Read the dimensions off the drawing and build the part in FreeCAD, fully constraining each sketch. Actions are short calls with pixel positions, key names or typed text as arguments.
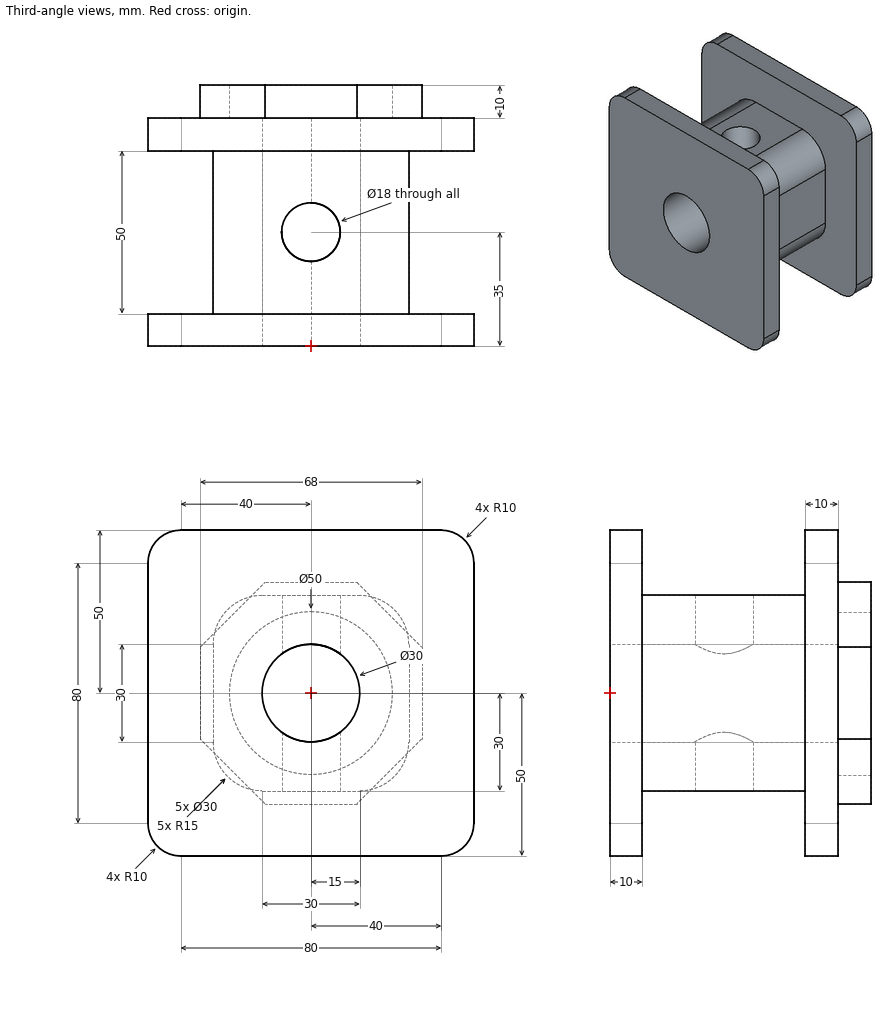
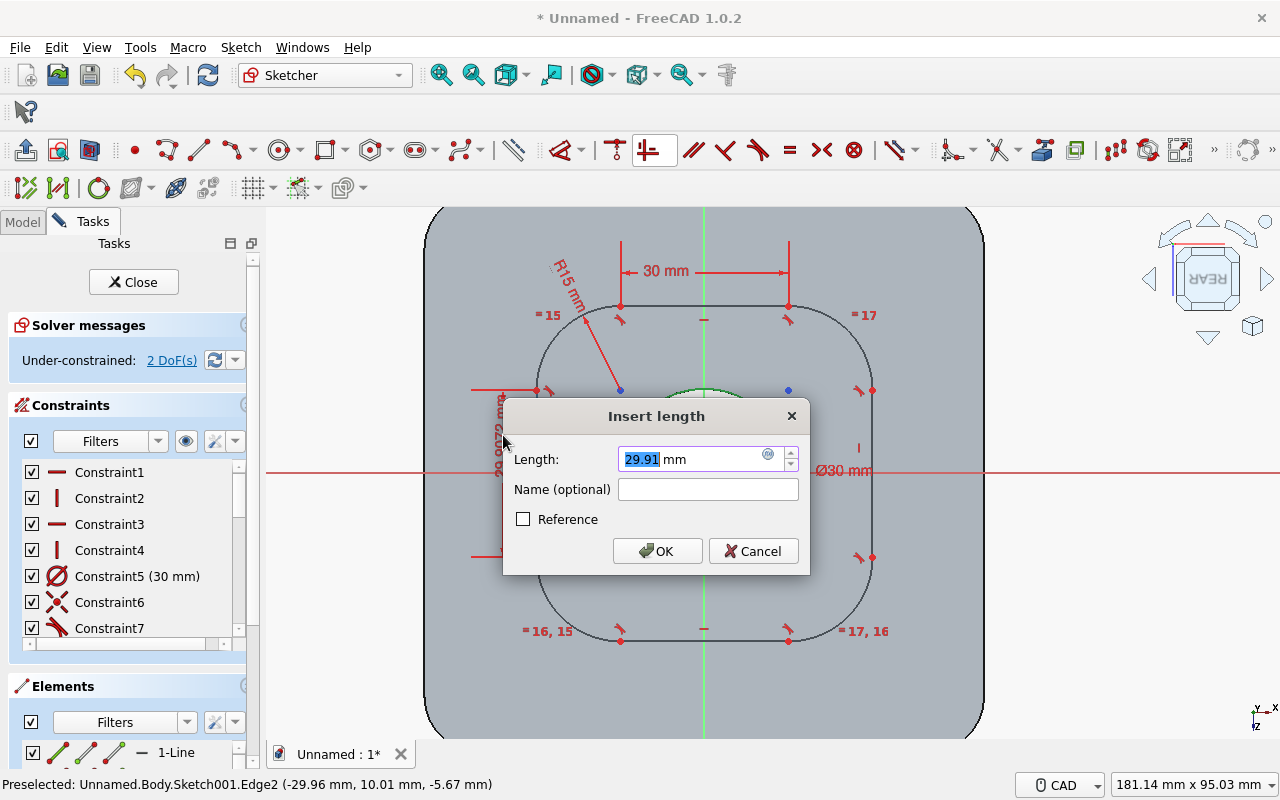
text(30)
key(Return)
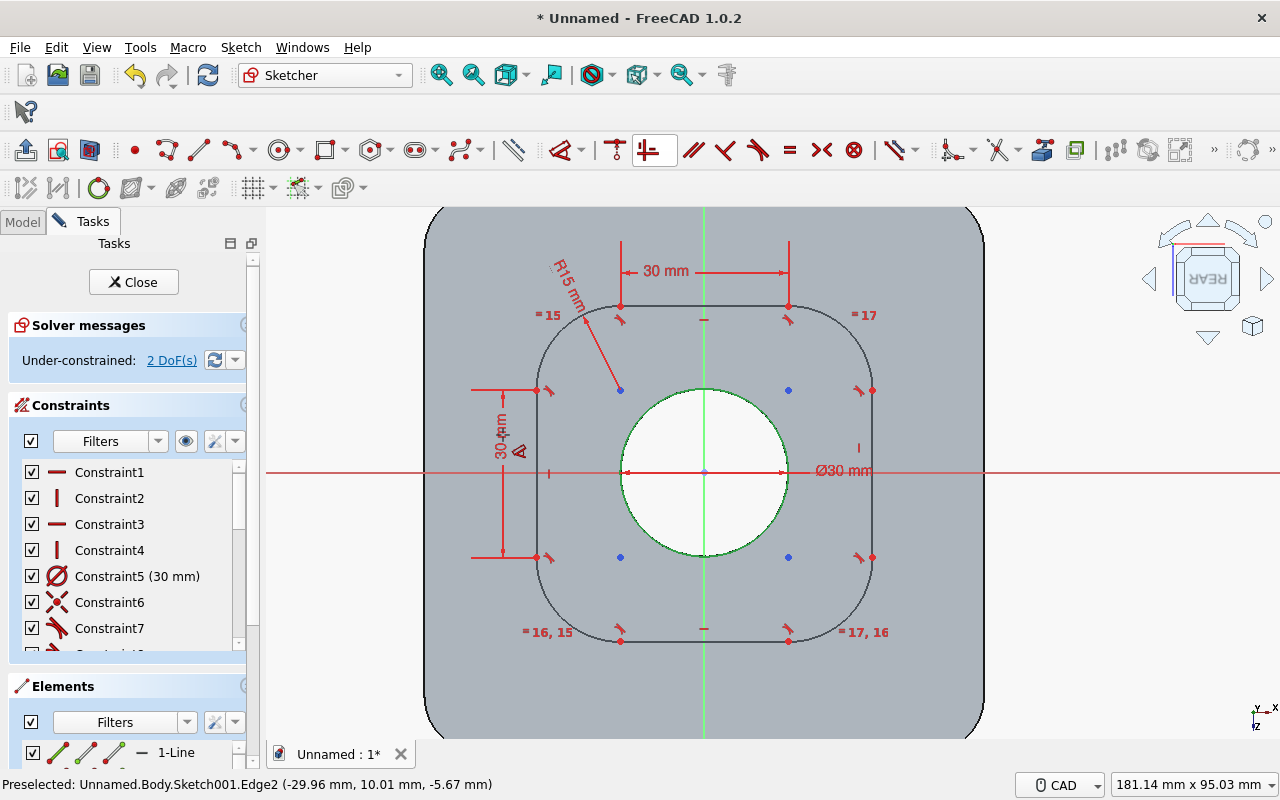
click(789, 306)
click(746, 272)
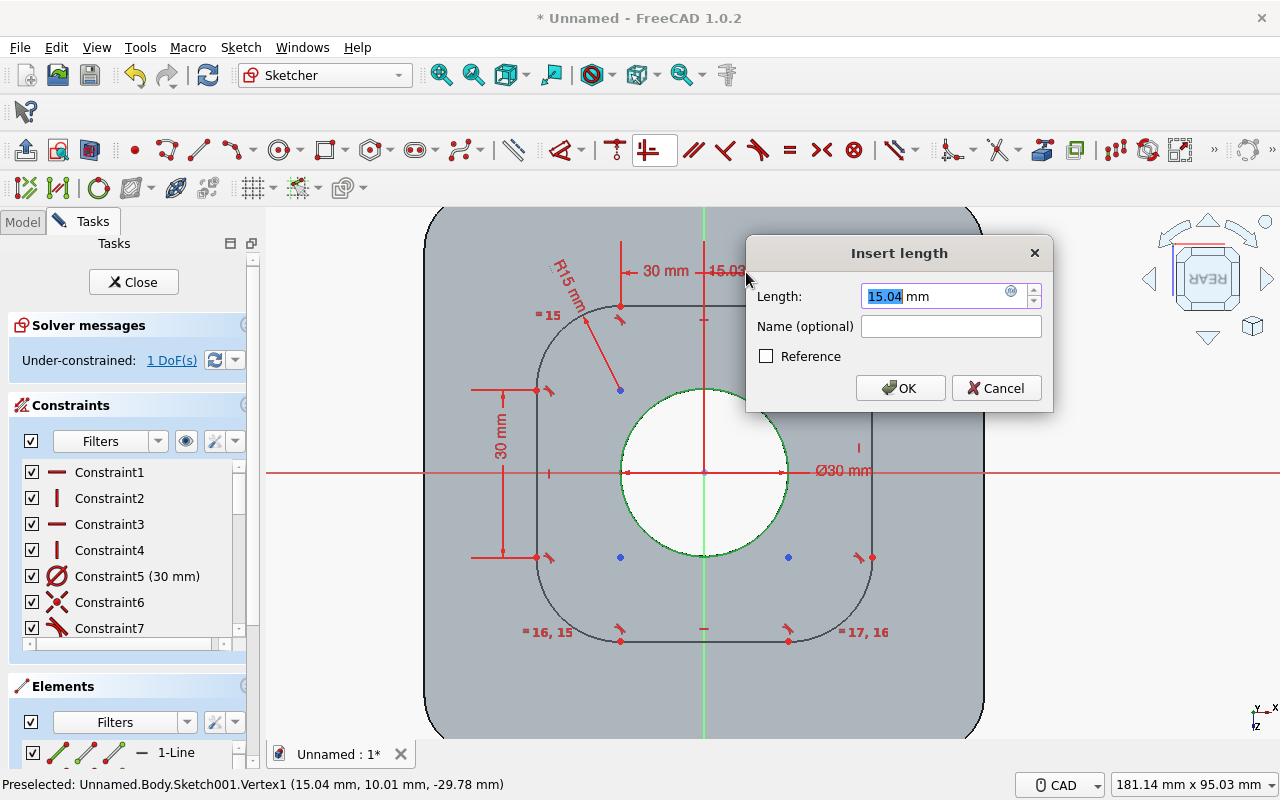
text(15)
key(Return)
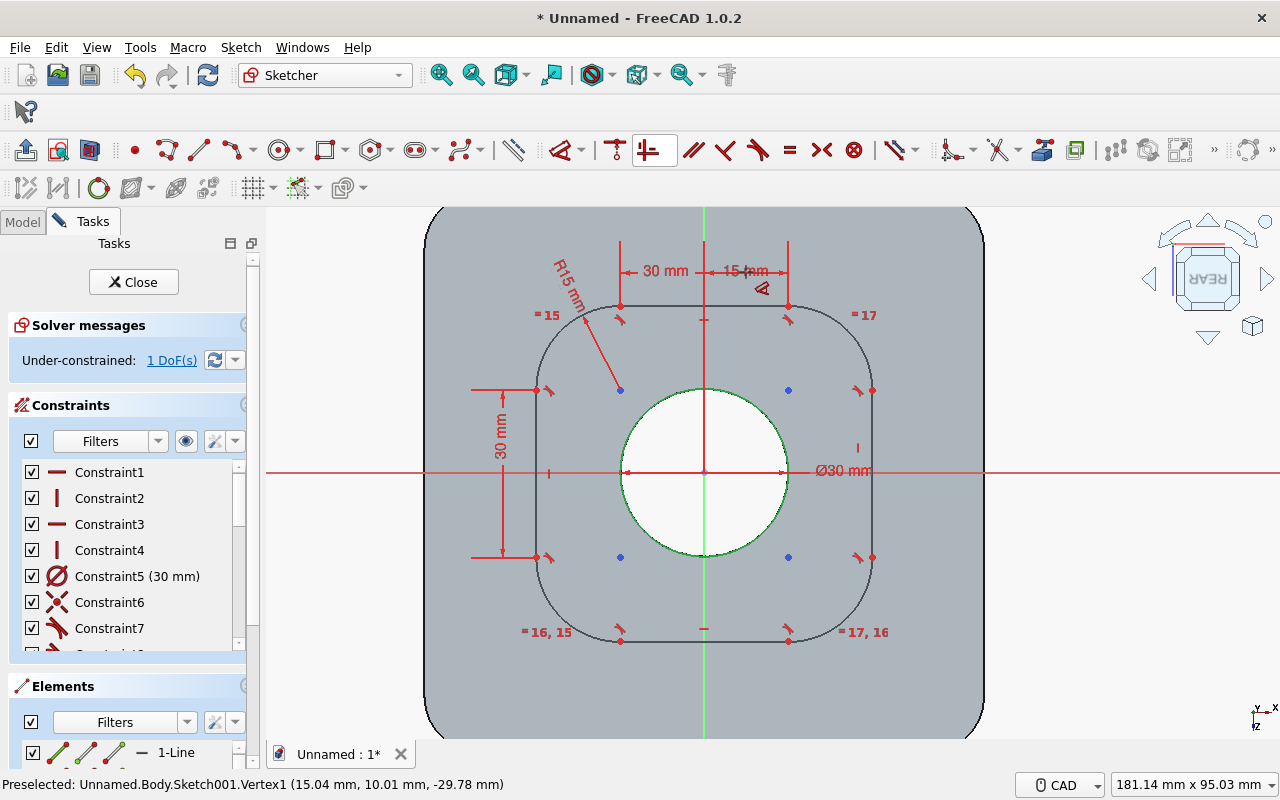
click(788, 306)
click(822, 389)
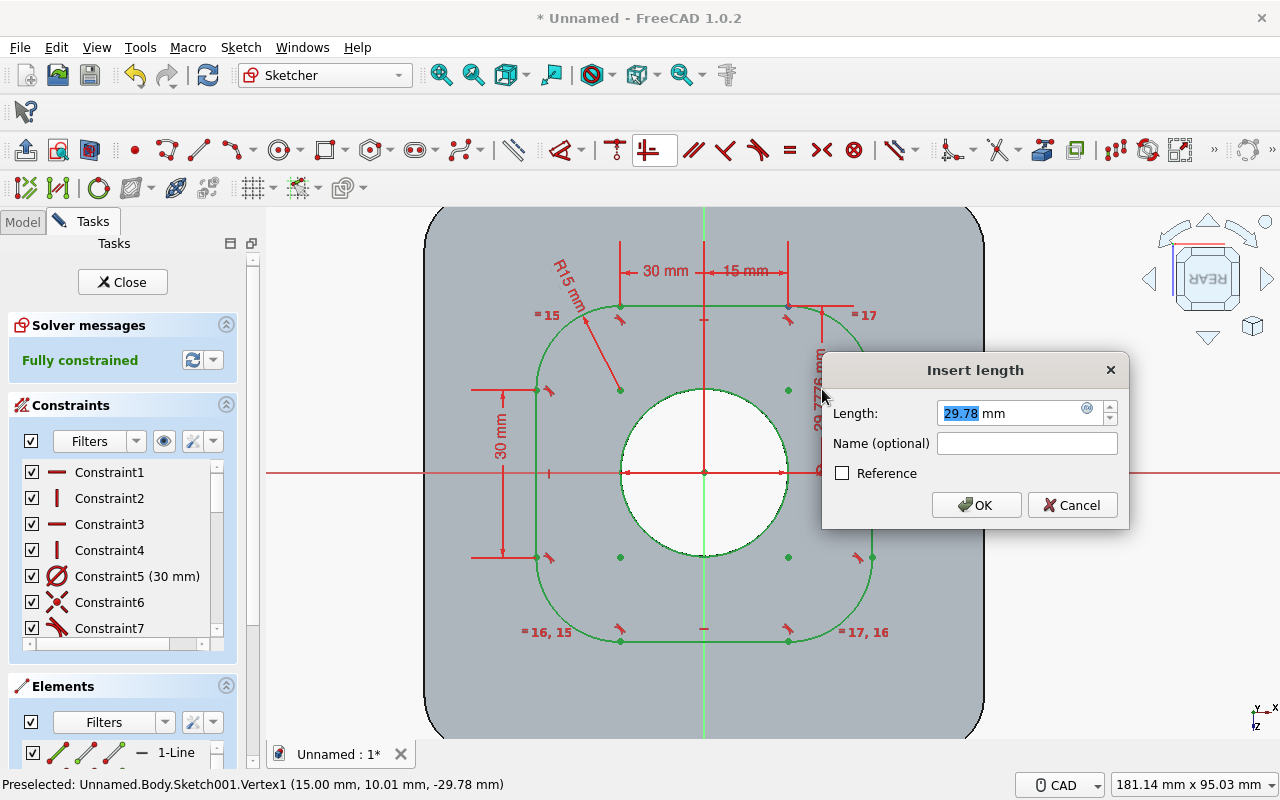
text(30)
key(Return)
key(Escape)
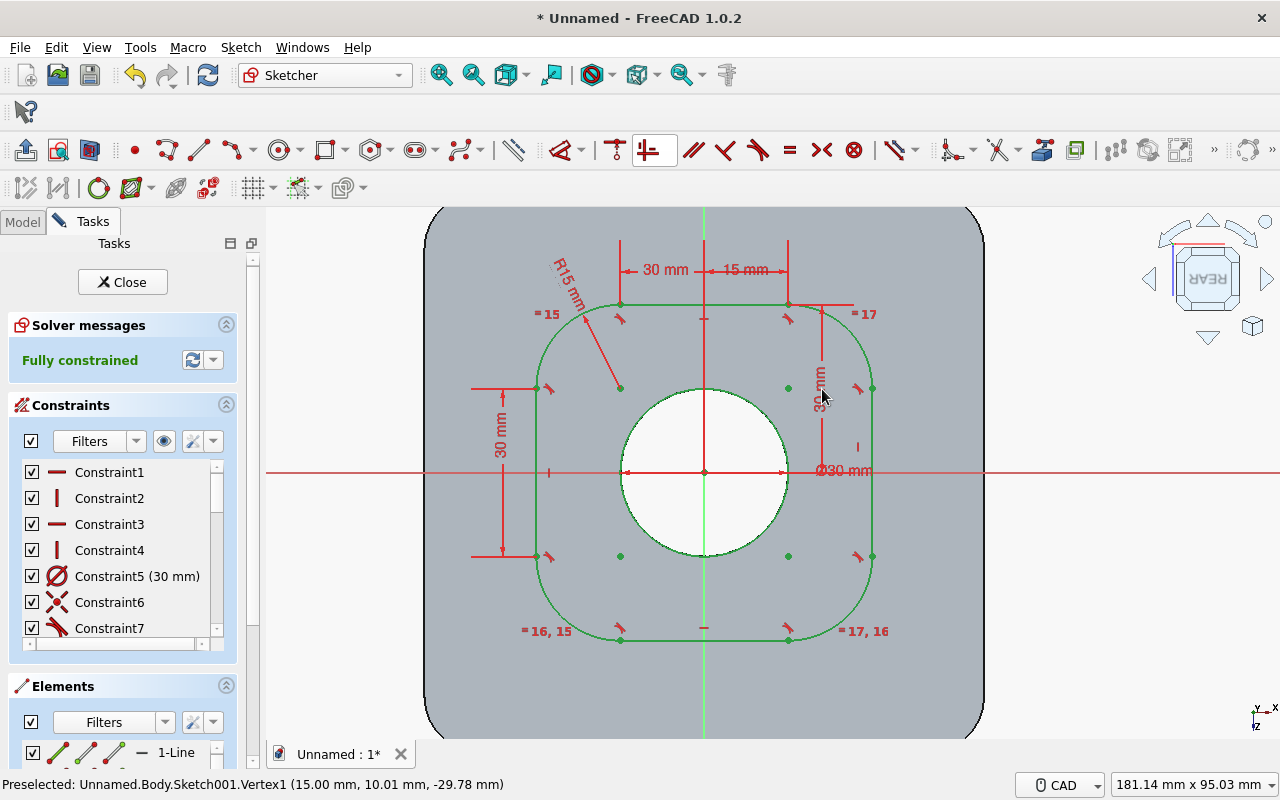
click(123, 282)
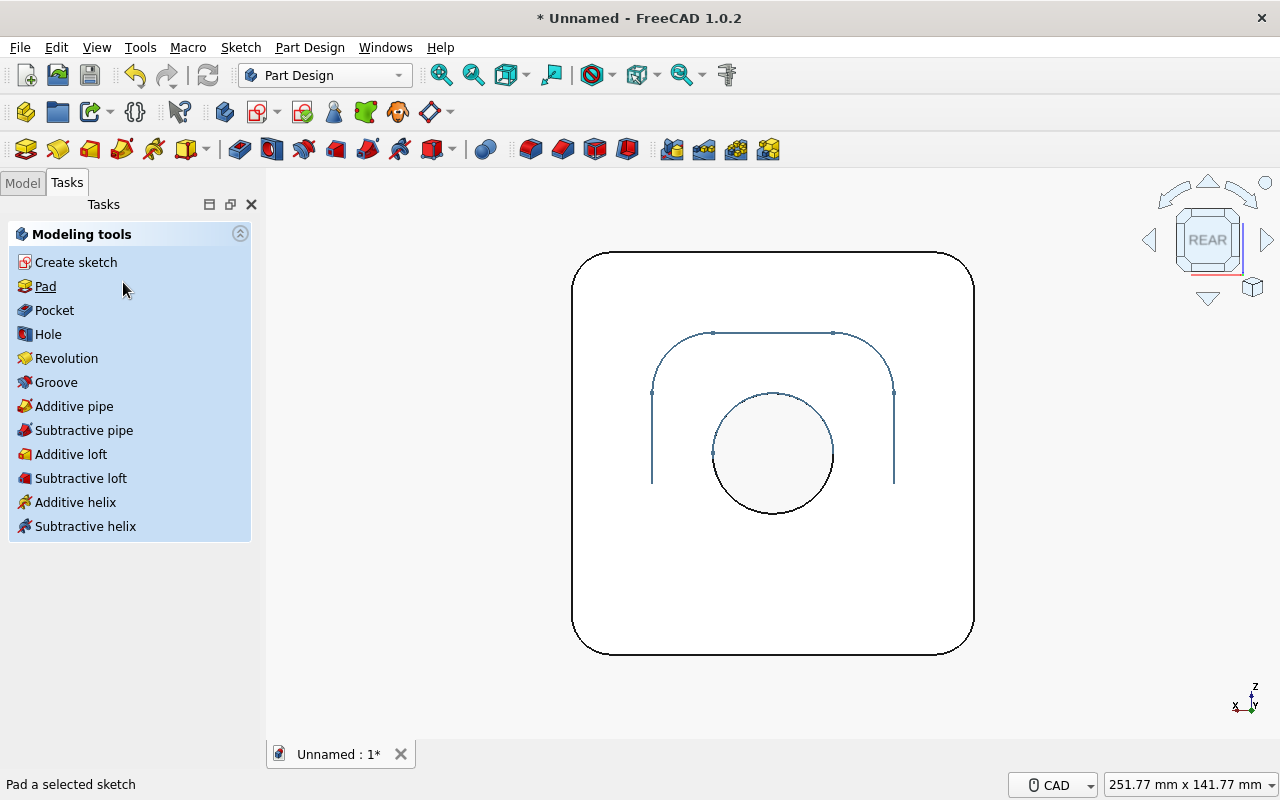
click(26, 150)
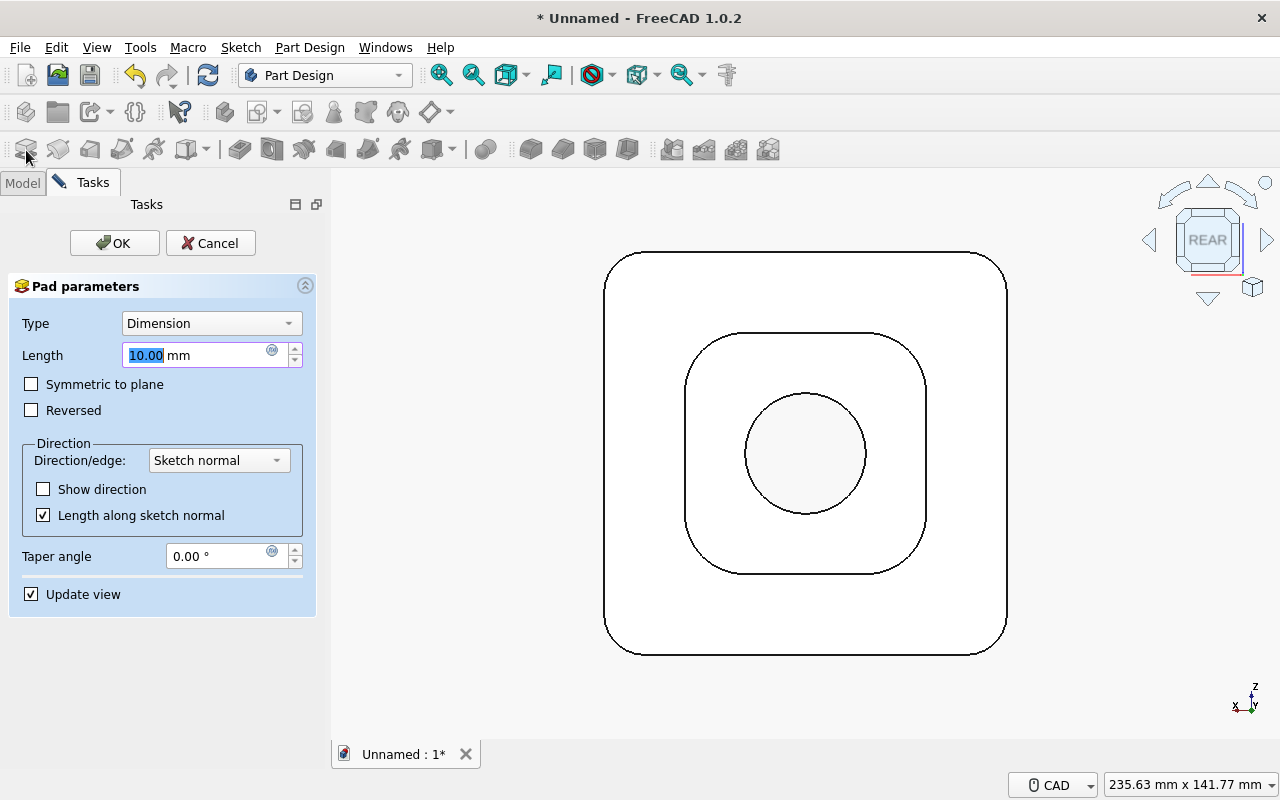
text(50)
key(Tab)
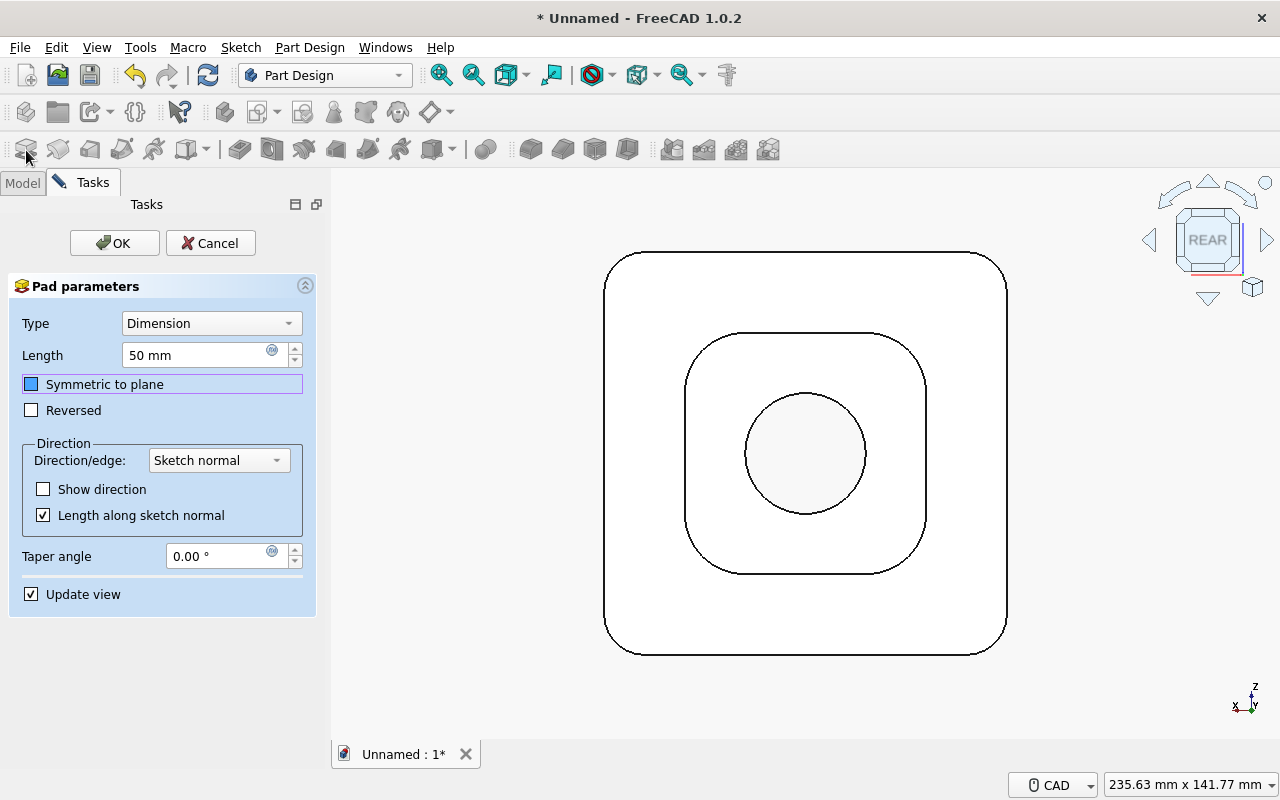
click(115, 243)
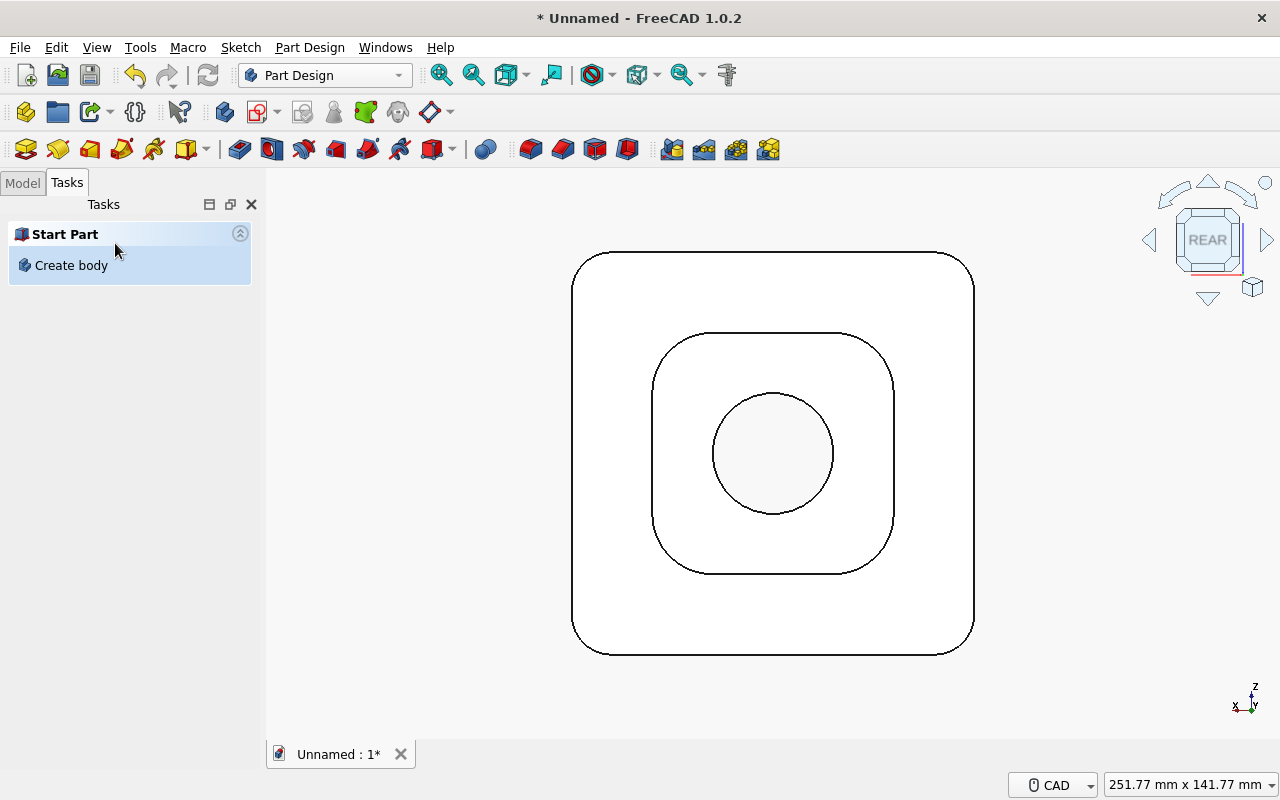
click(704, 522)